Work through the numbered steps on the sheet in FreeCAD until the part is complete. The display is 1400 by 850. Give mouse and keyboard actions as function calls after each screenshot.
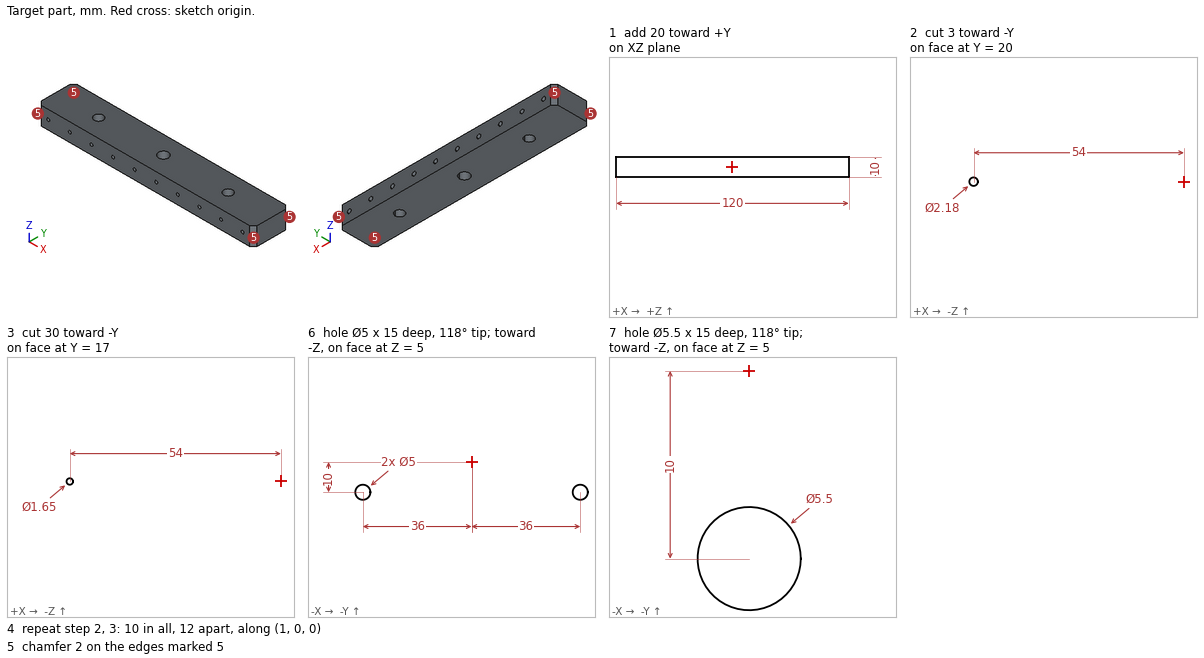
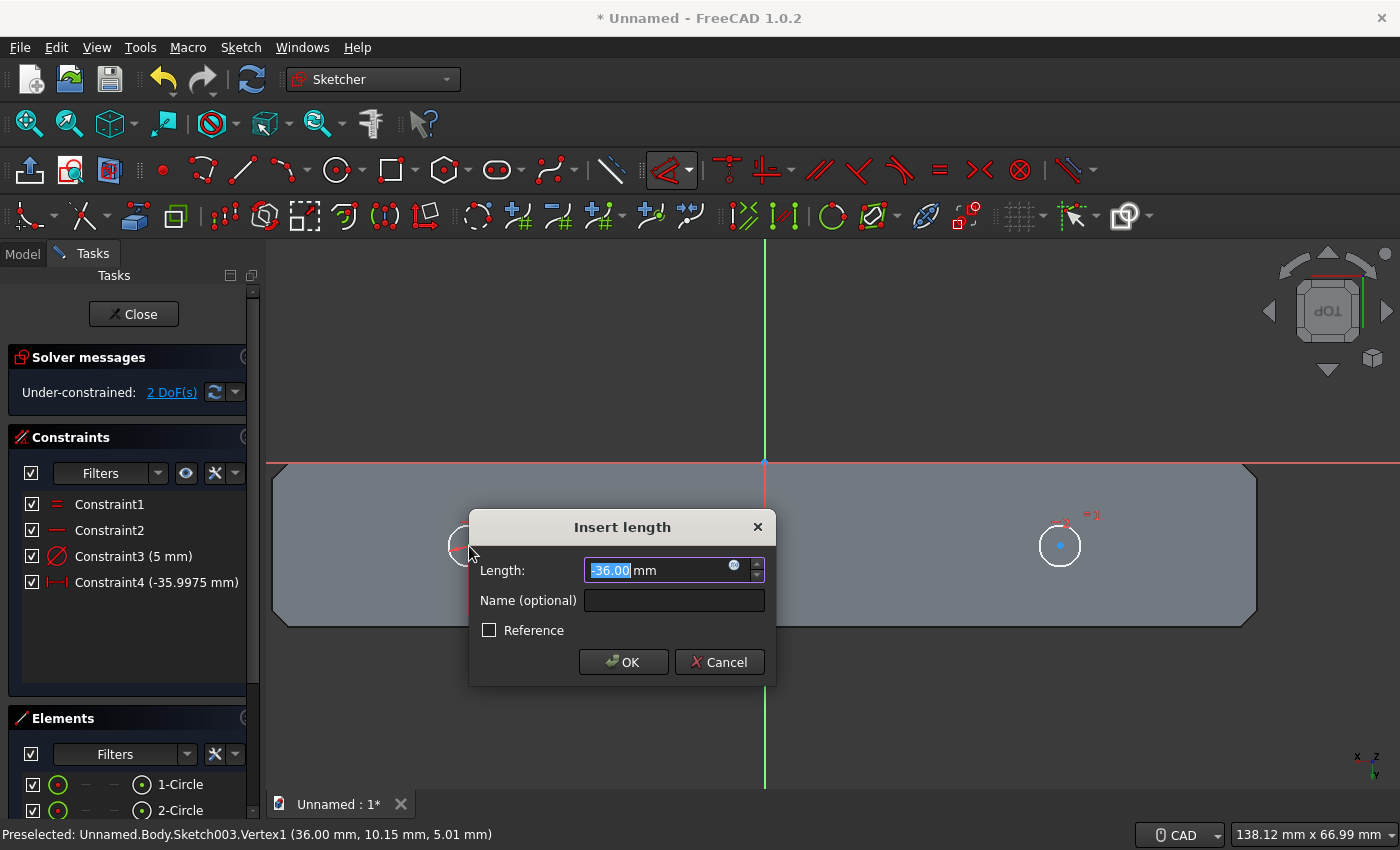
text(-36)
key(Return)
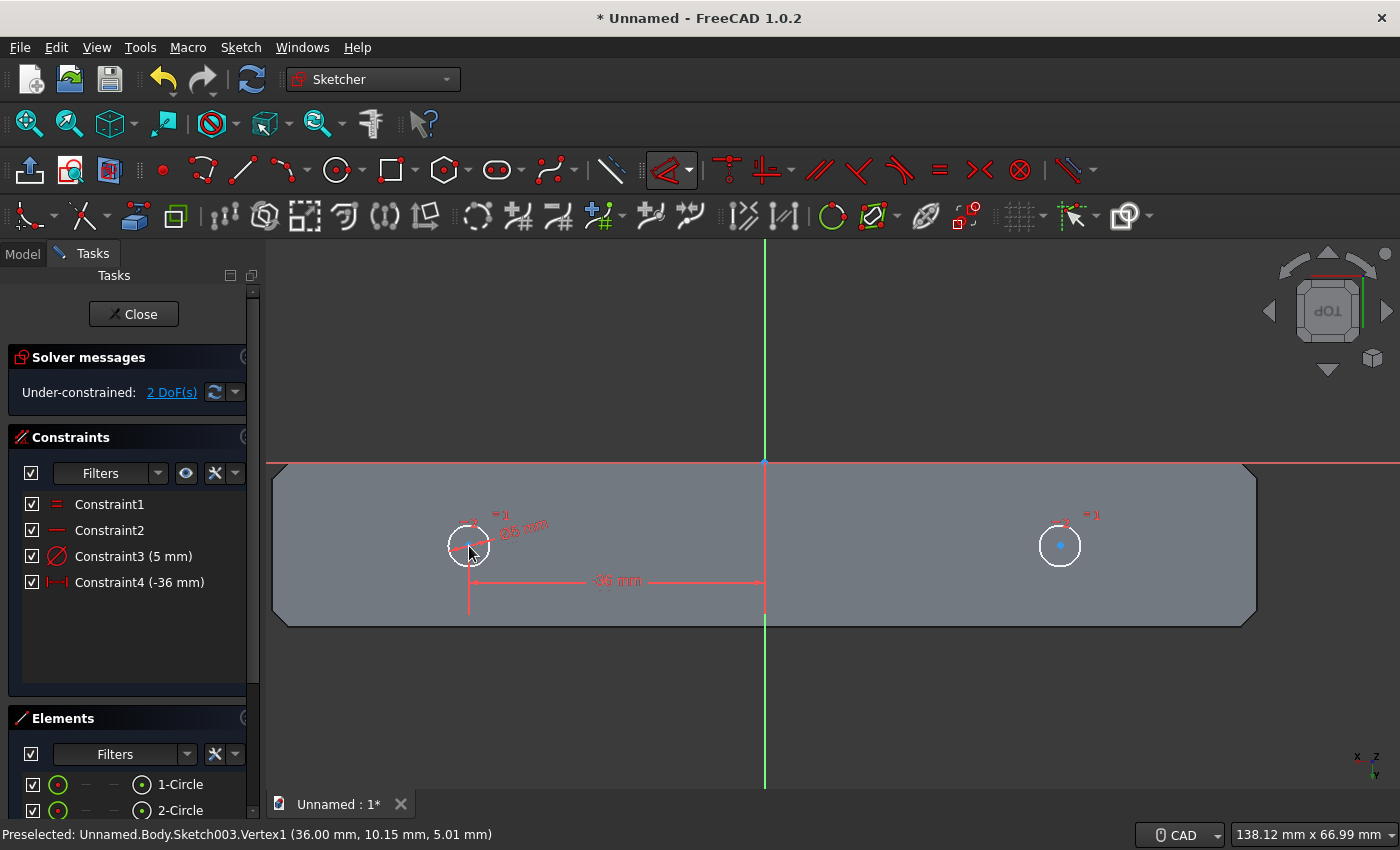
click(469, 546)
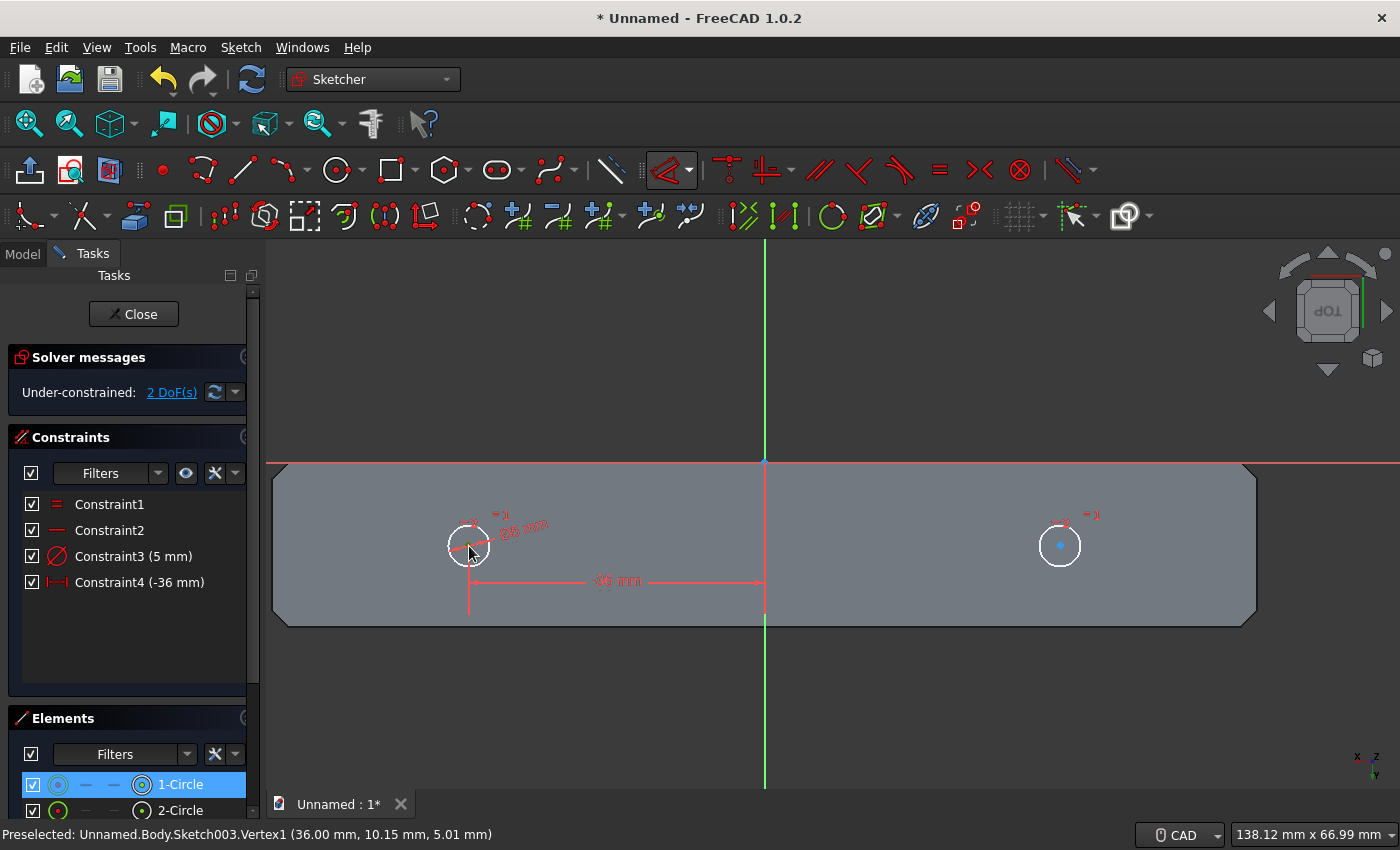
click(692, 170)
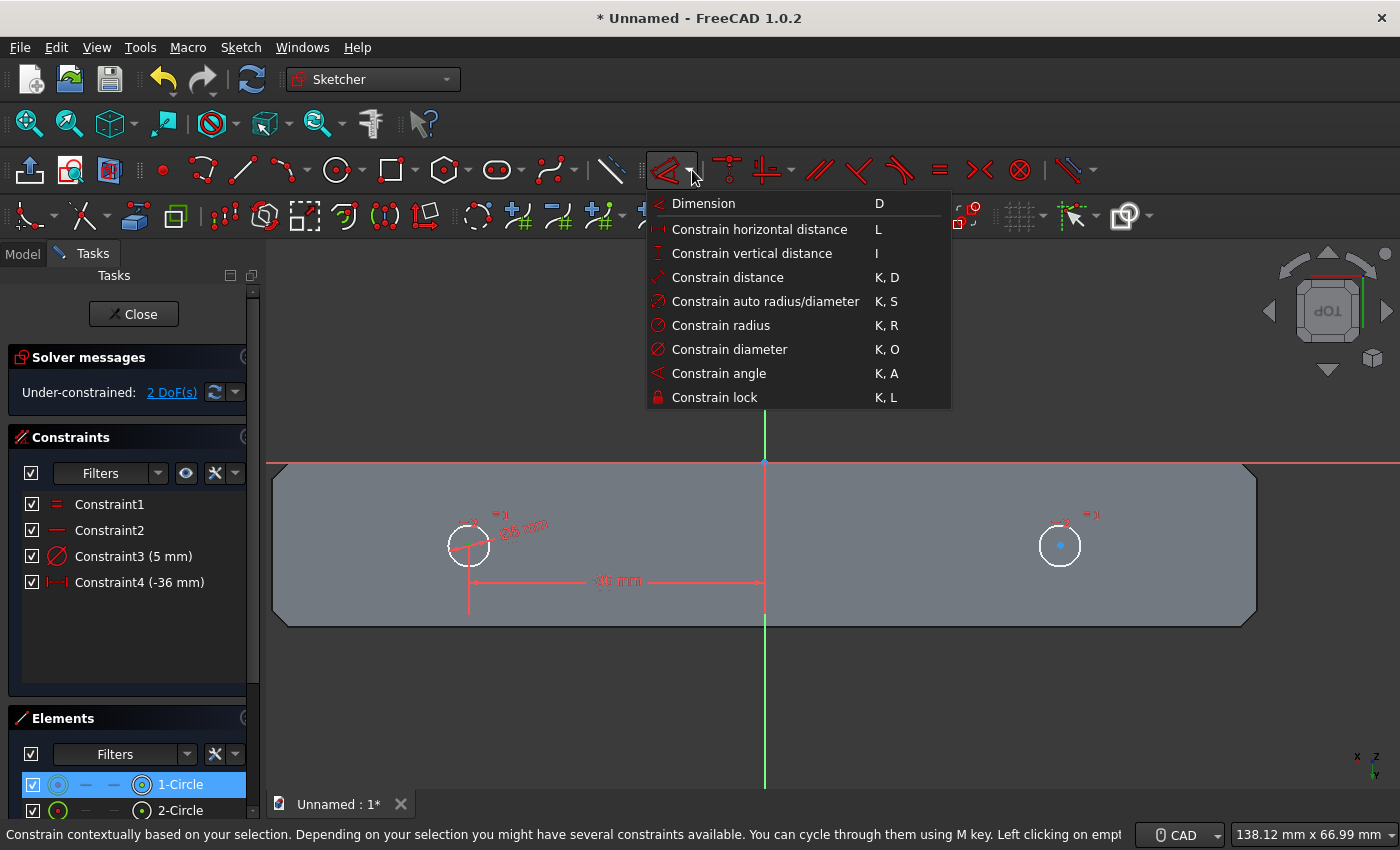
click(799, 253)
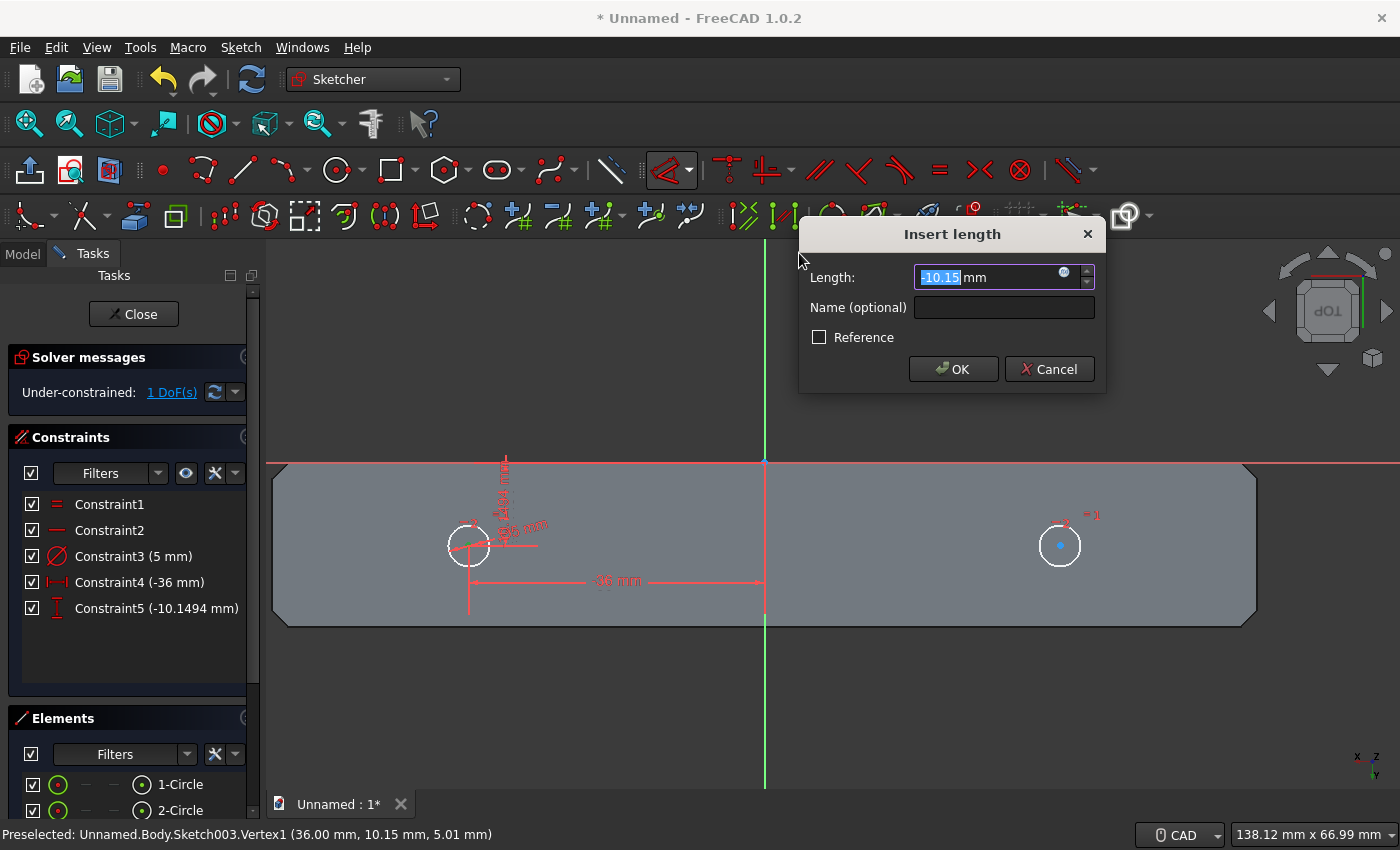
text(-10)
key(Return)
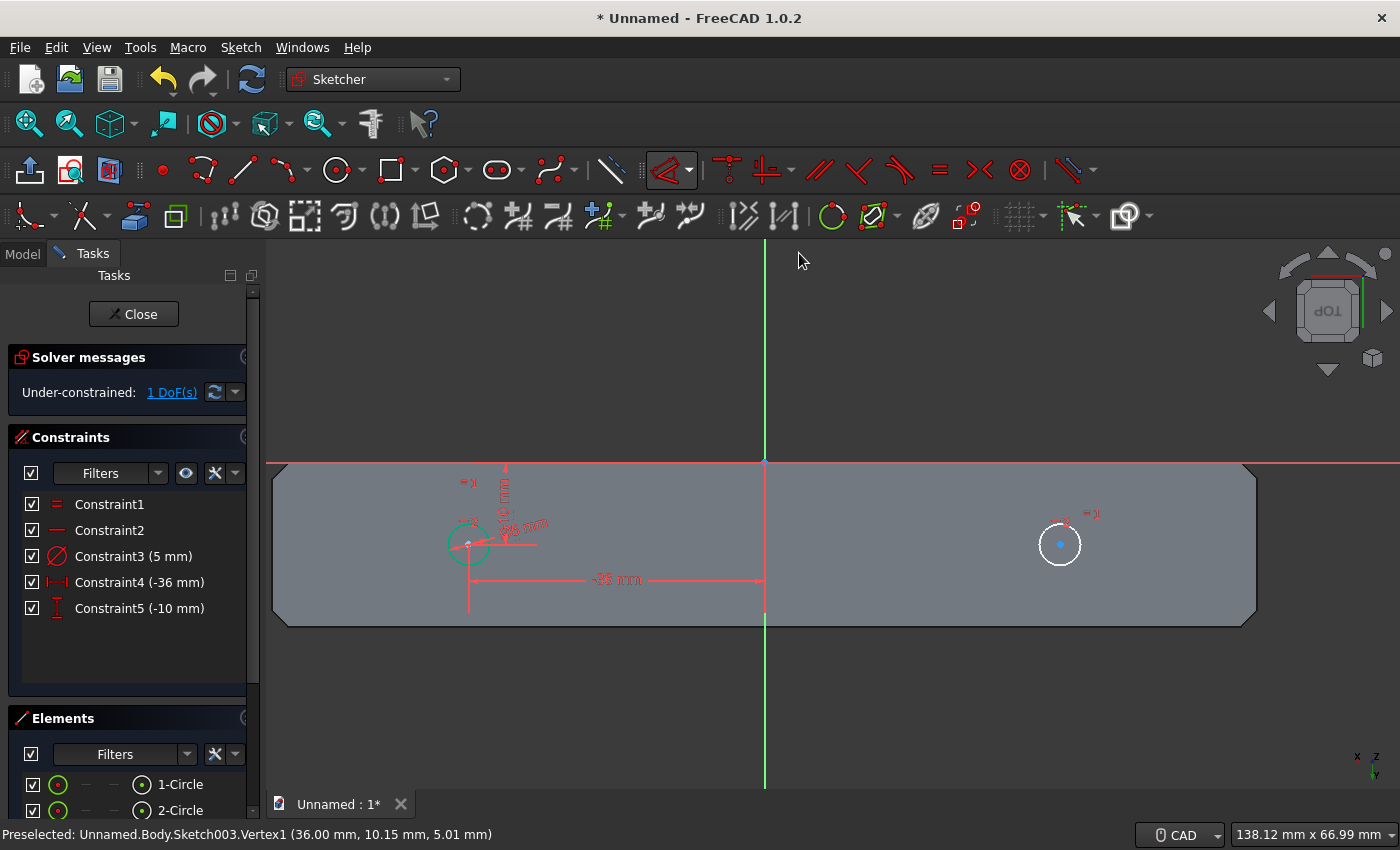
click(1060, 545)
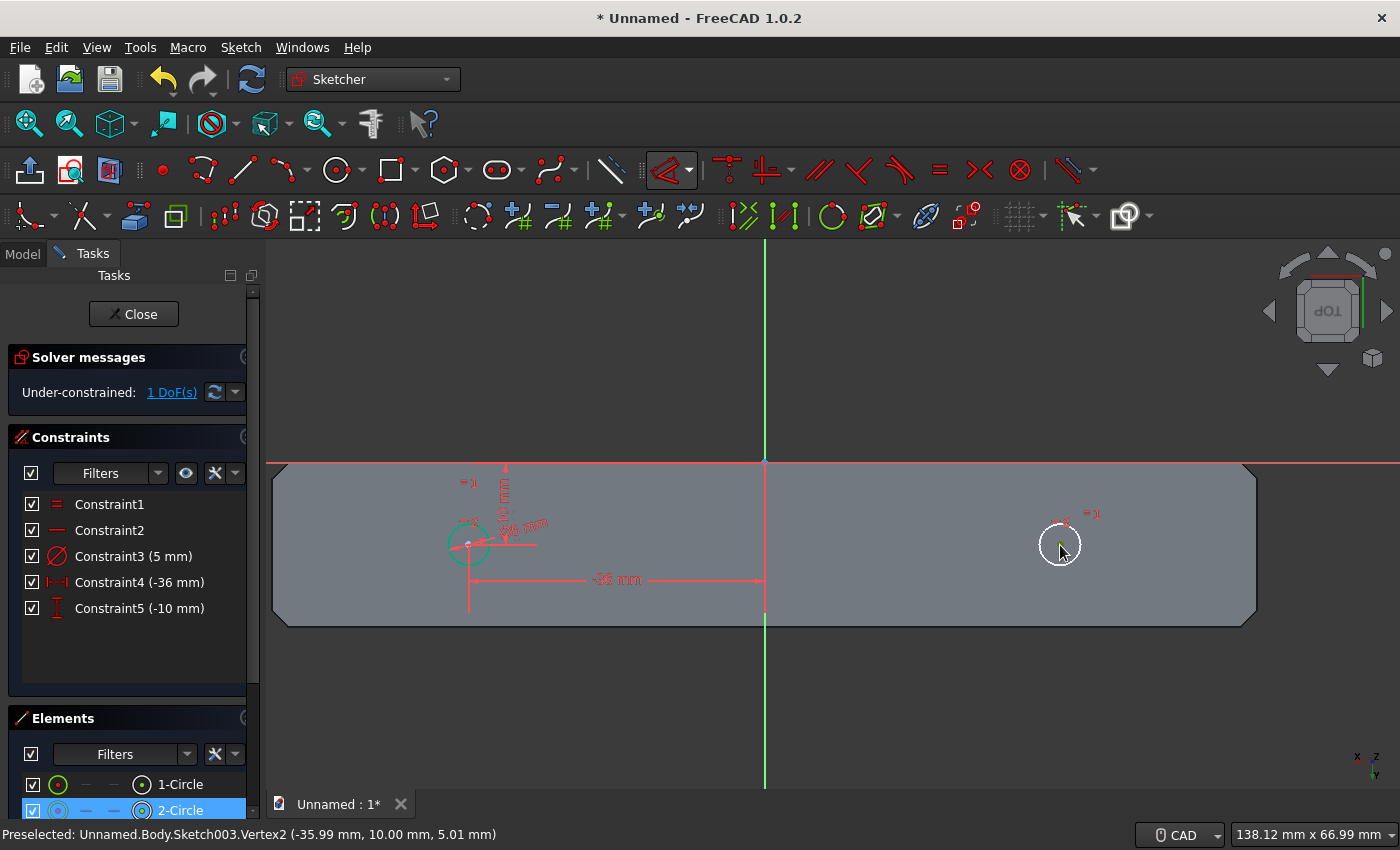
click(692, 170)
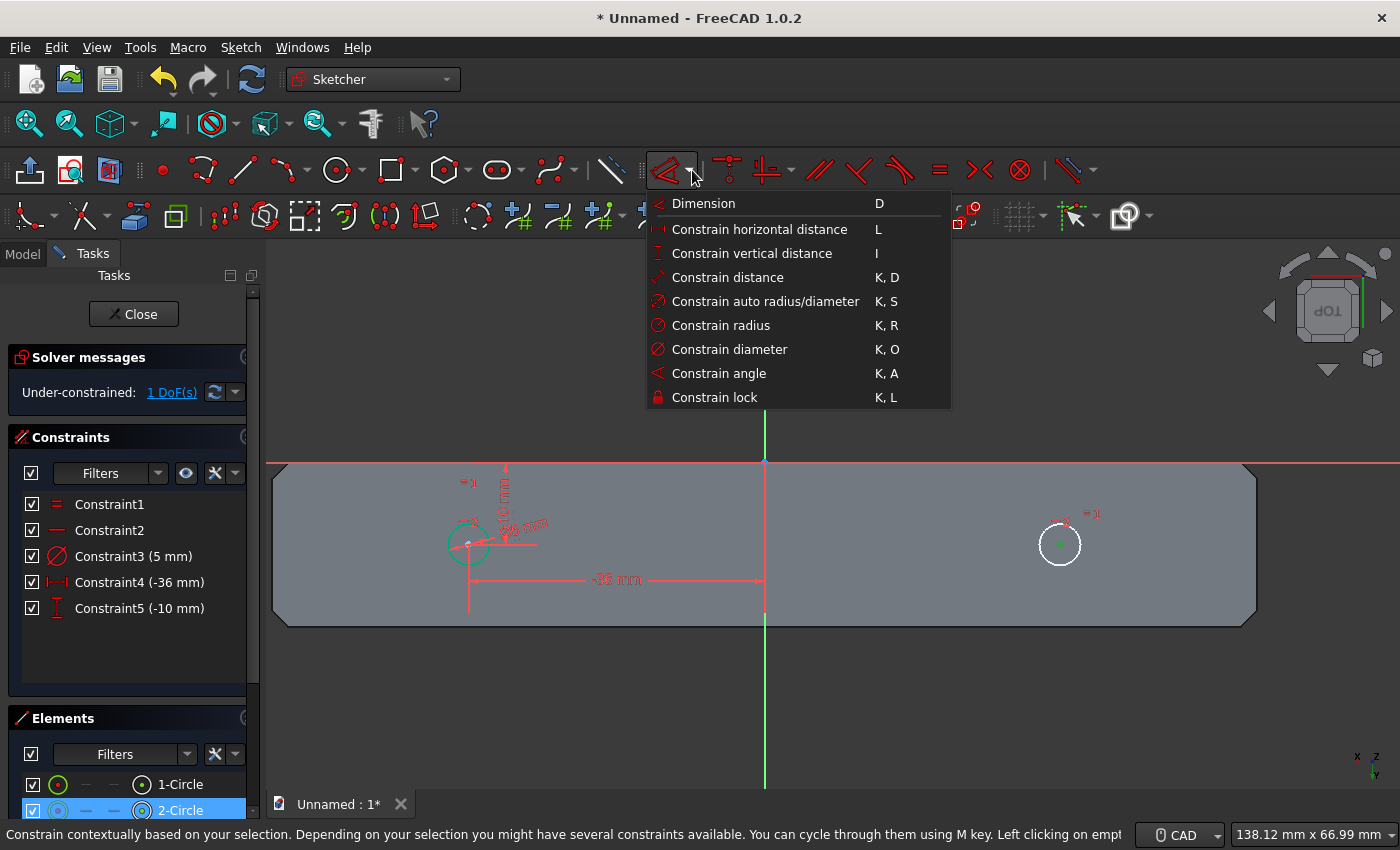
click(799, 229)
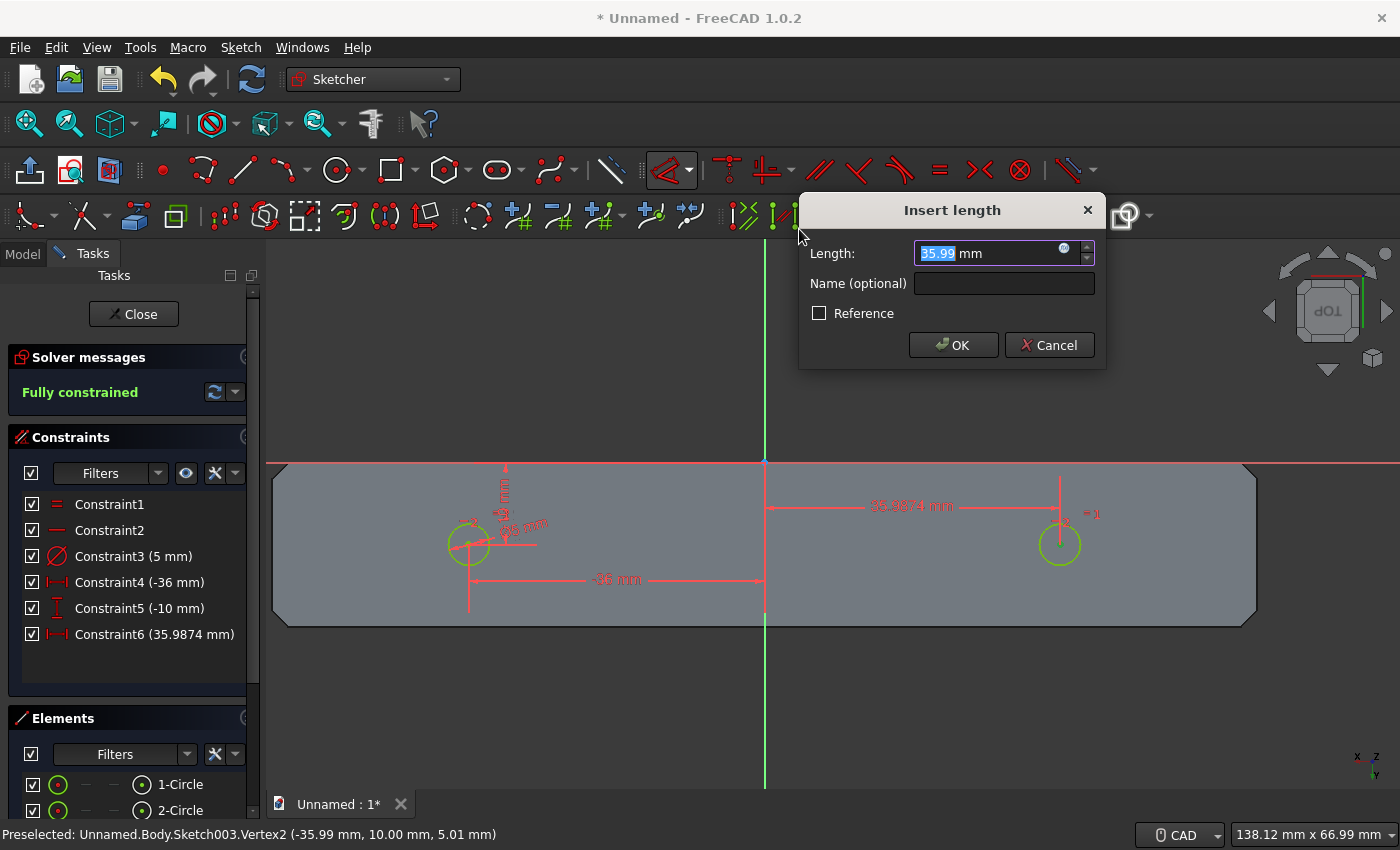
text(36)
key(Return)